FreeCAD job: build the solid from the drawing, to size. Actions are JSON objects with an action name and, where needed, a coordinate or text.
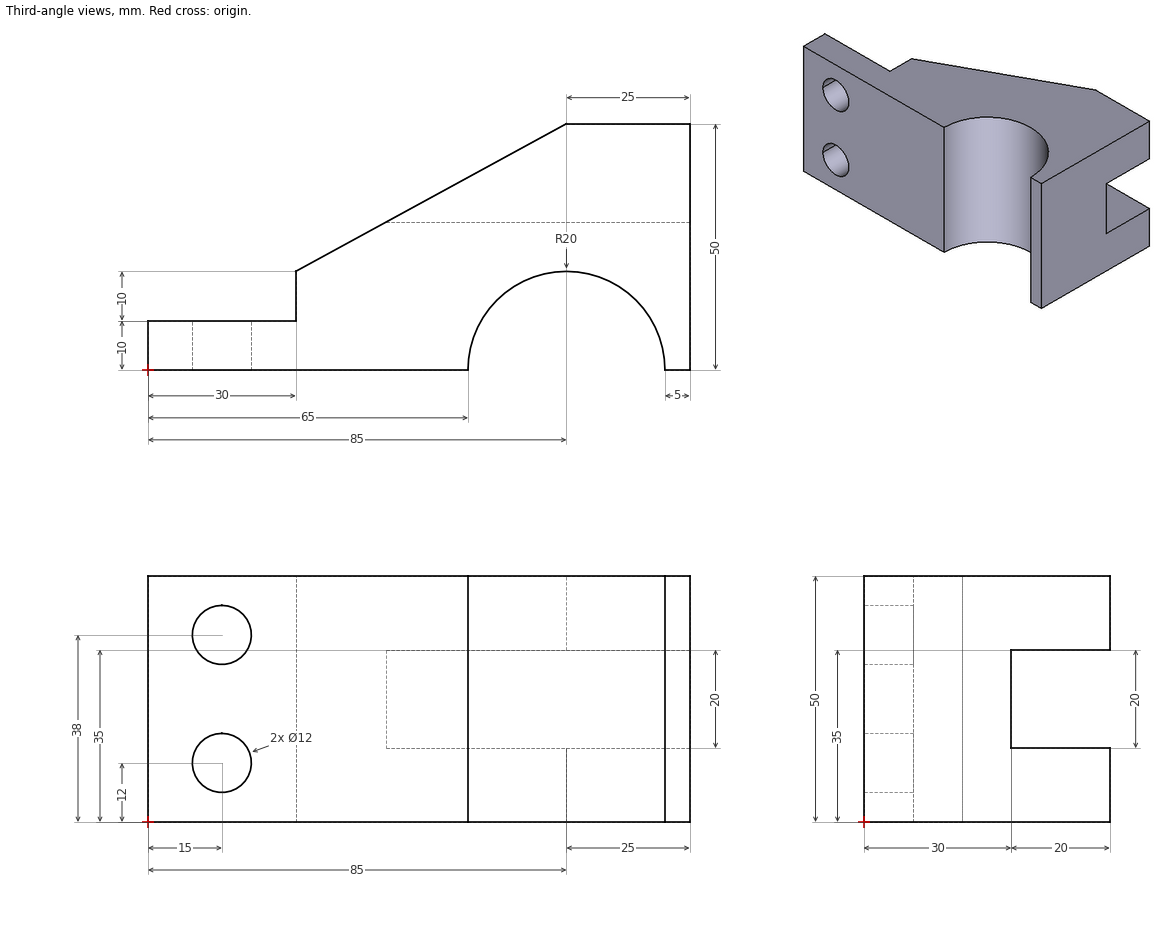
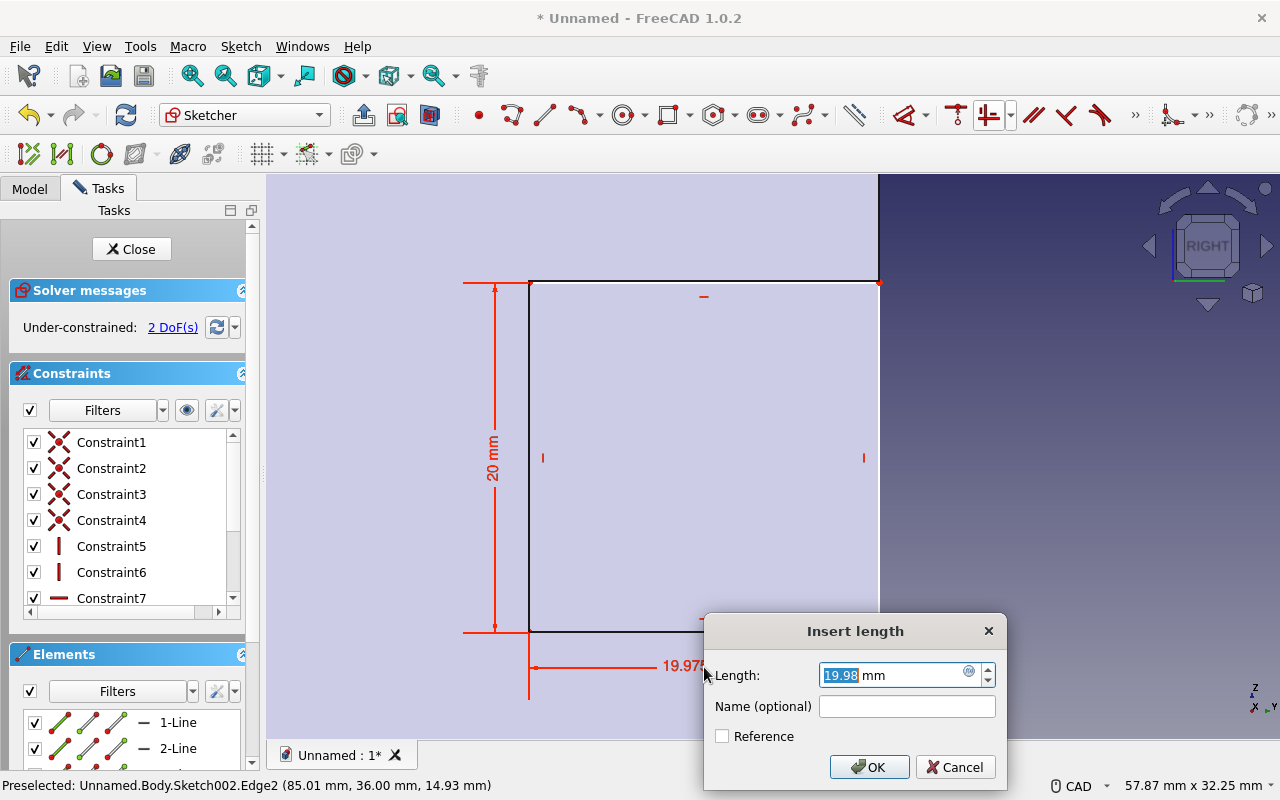
{"action": "type", "text": "20"}
{"action": "key", "text": "Return"}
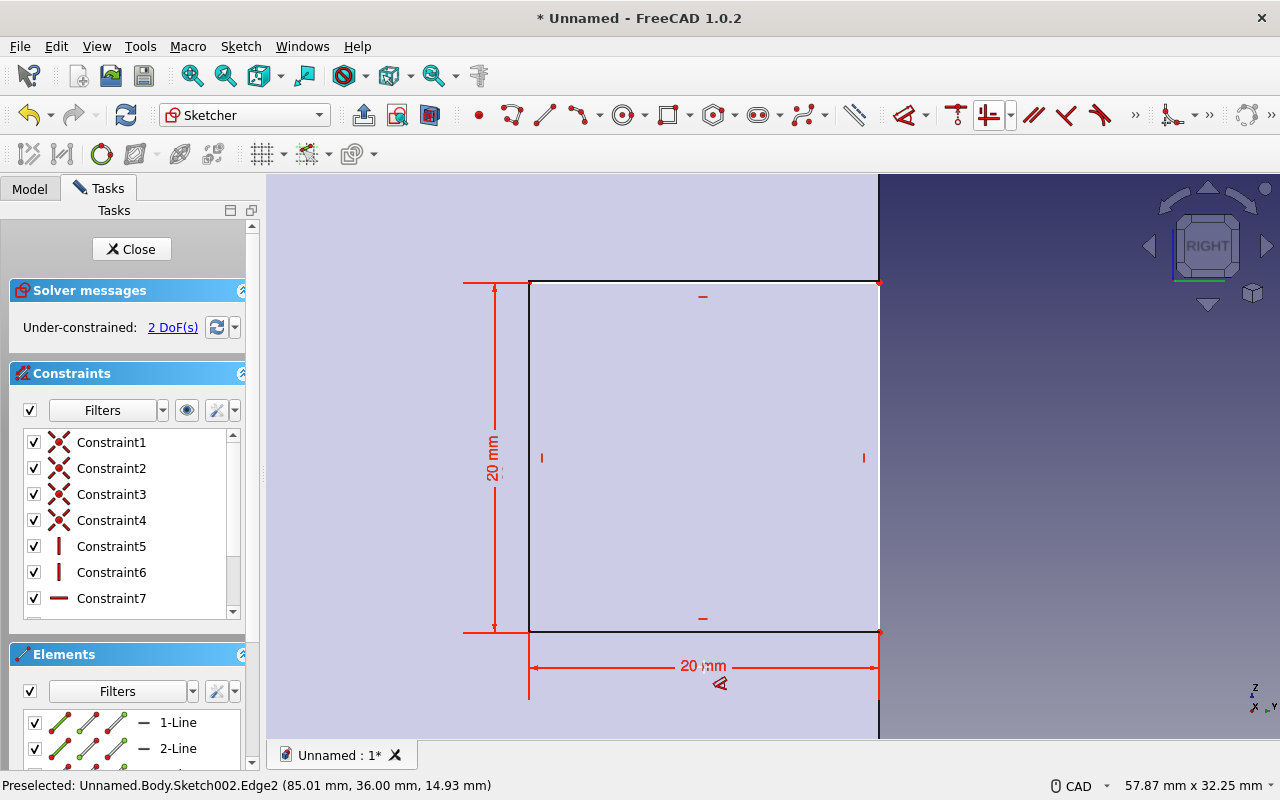
{"action": "left_click", "coordinate": [529, 283]}
{"action": "left_click", "coordinate": [411, 249]}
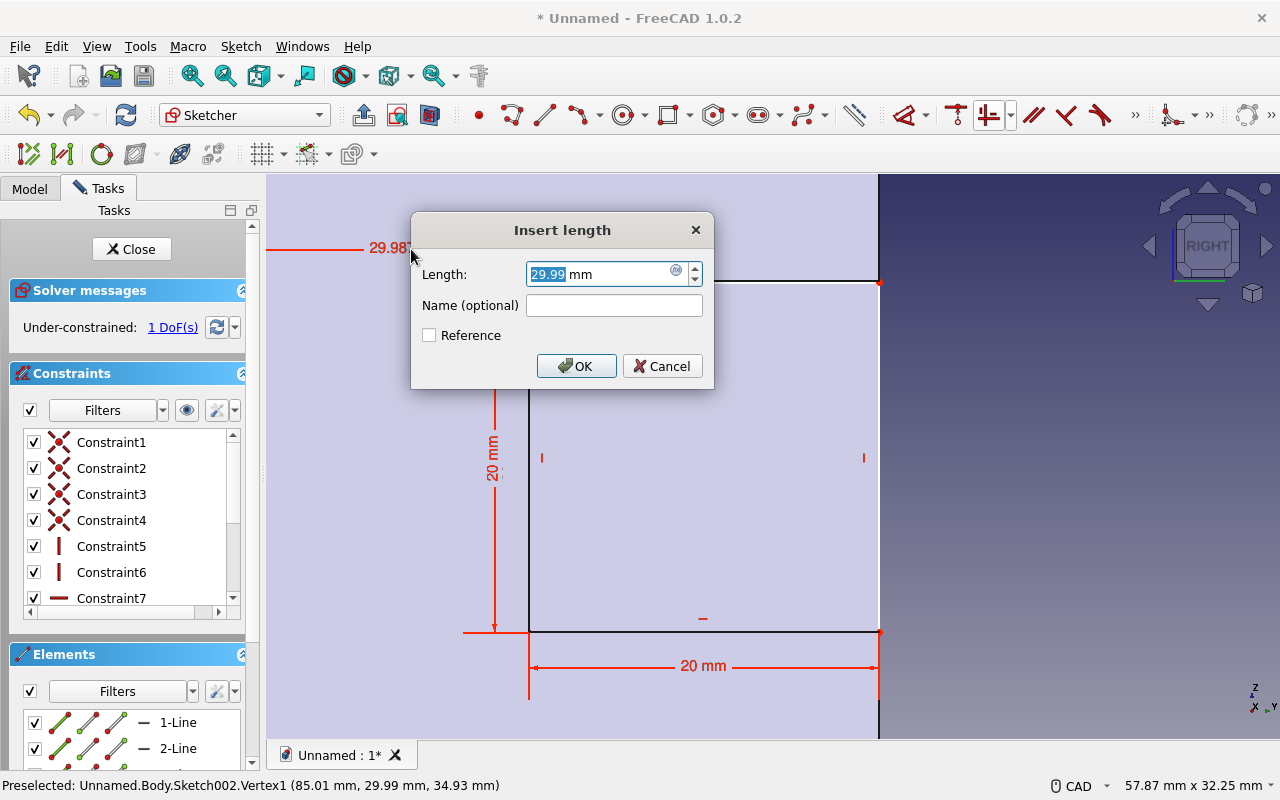
{"action": "type", "text": "30"}
{"action": "key", "text": "Return"}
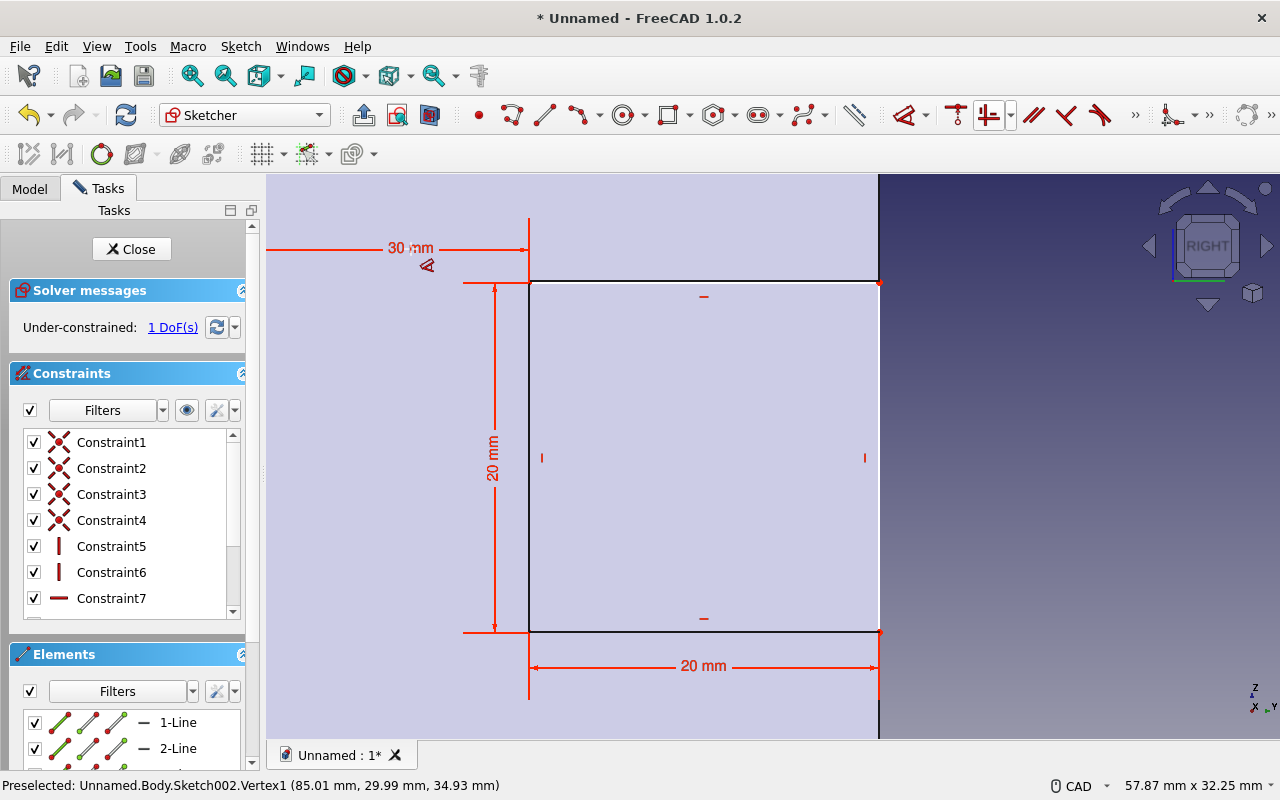
{"action": "left_click", "coordinate": [529, 283]}
{"action": "left_click", "coordinate": [563, 497]}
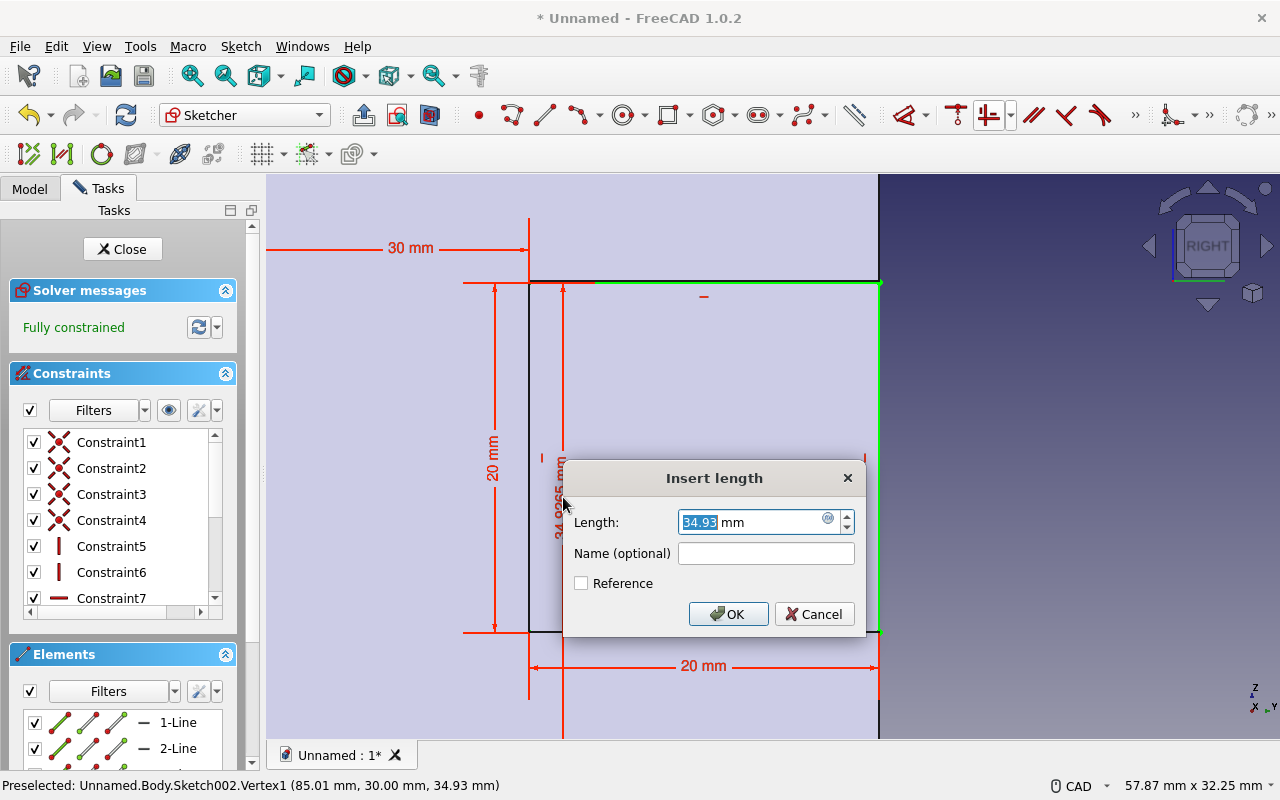
{"action": "type", "text": "35"}
{"action": "key", "text": "Return"}
{"action": "key", "text": "Escape"}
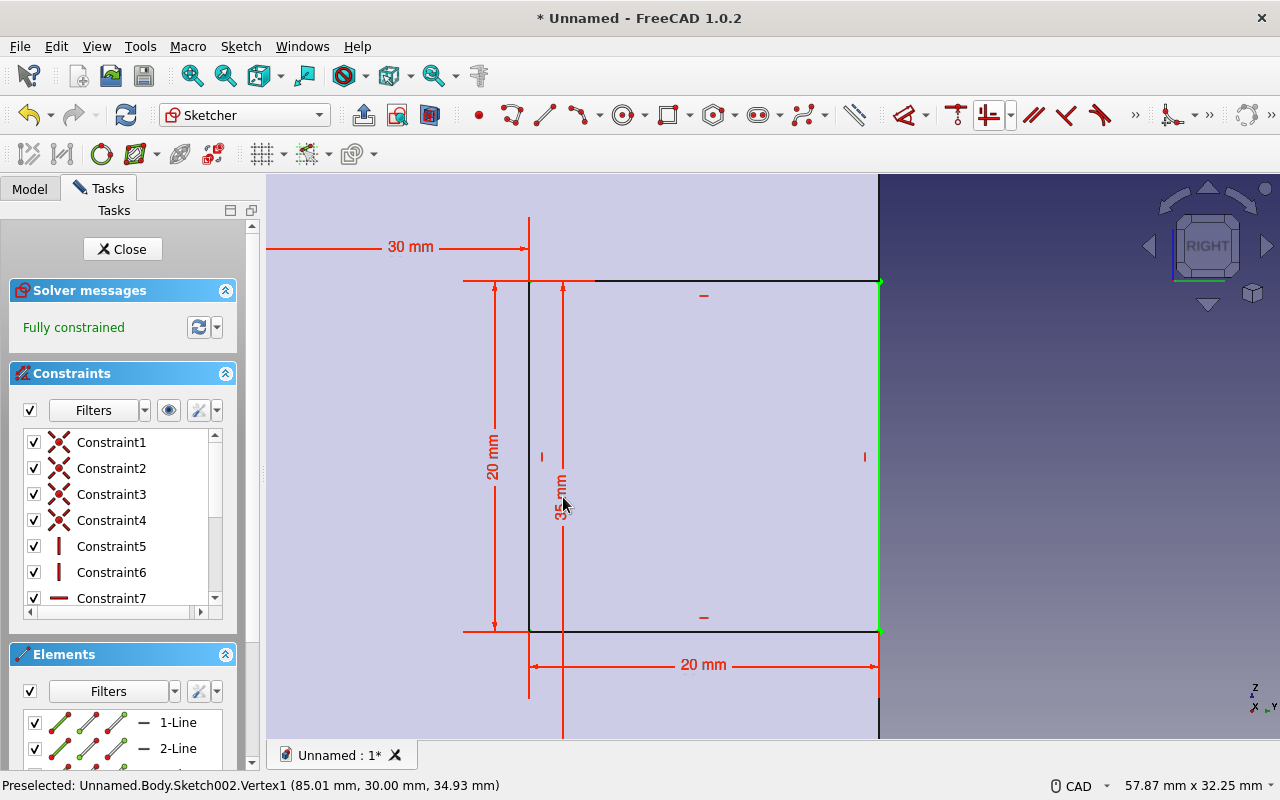
{"action": "left_click", "coordinate": [123, 249]}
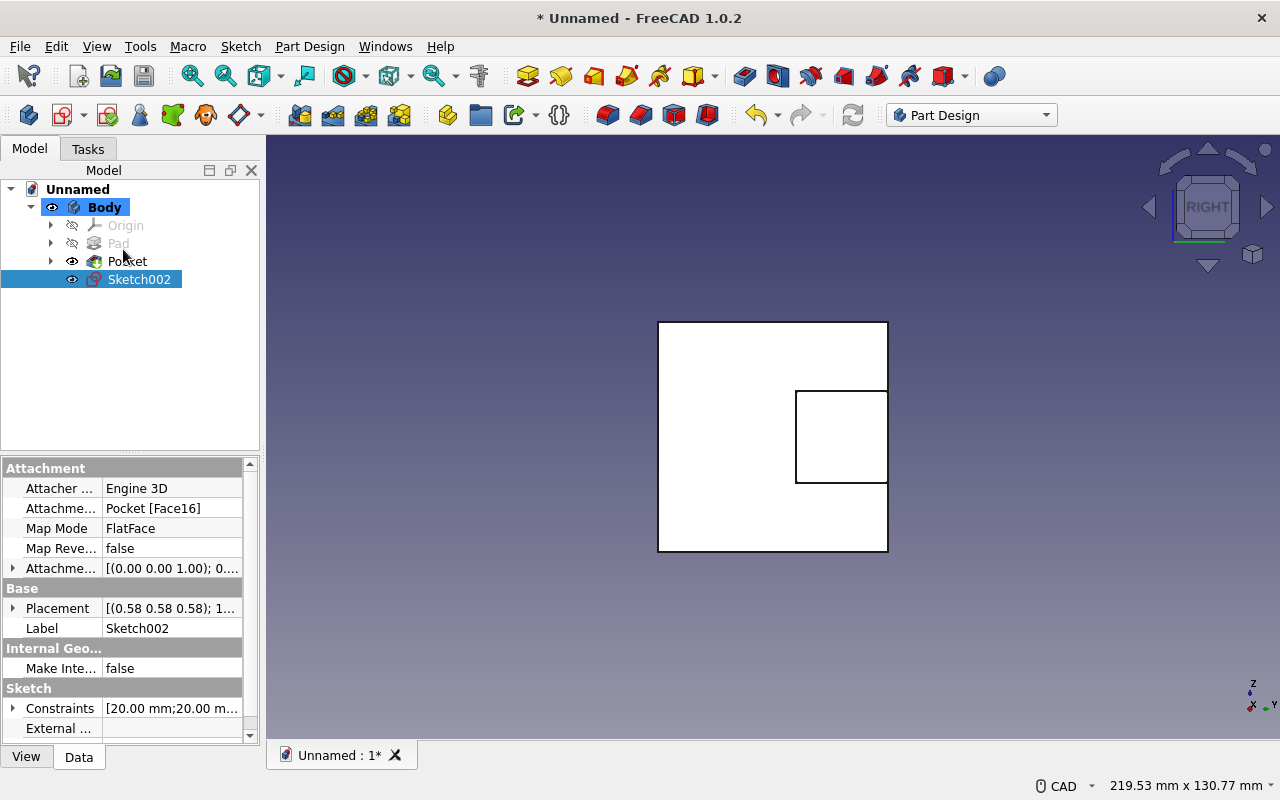
{"action": "left_click", "coordinate": [745, 76]}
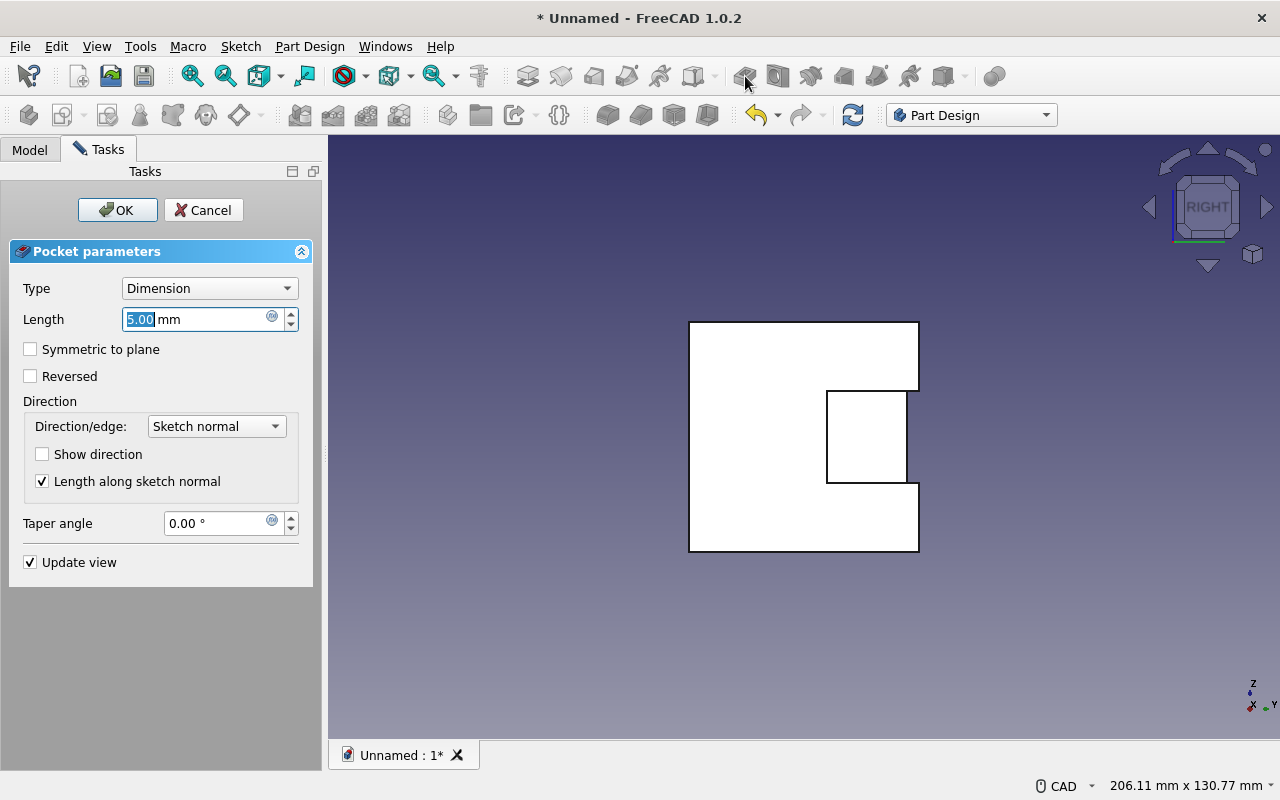
{"action": "left_click", "coordinate": [210, 288]}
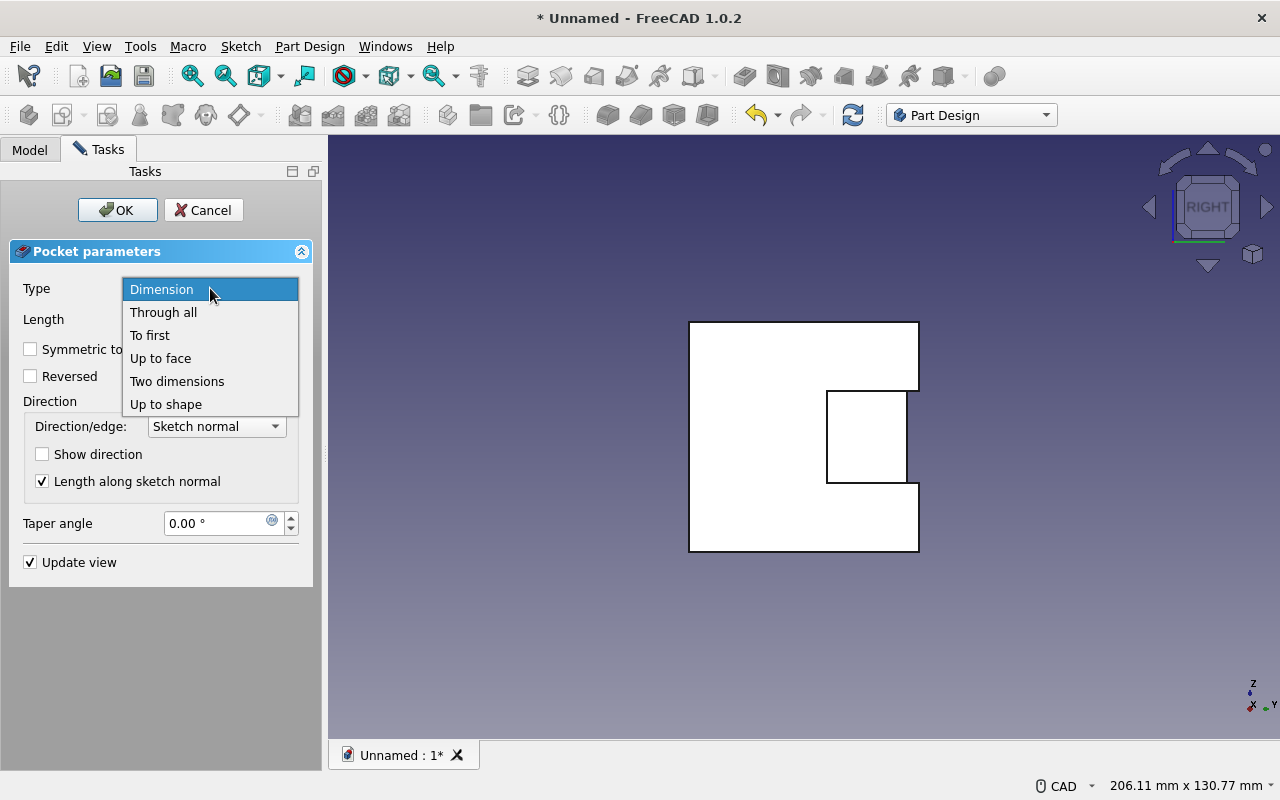
{"action": "left_click", "coordinate": [208, 312]}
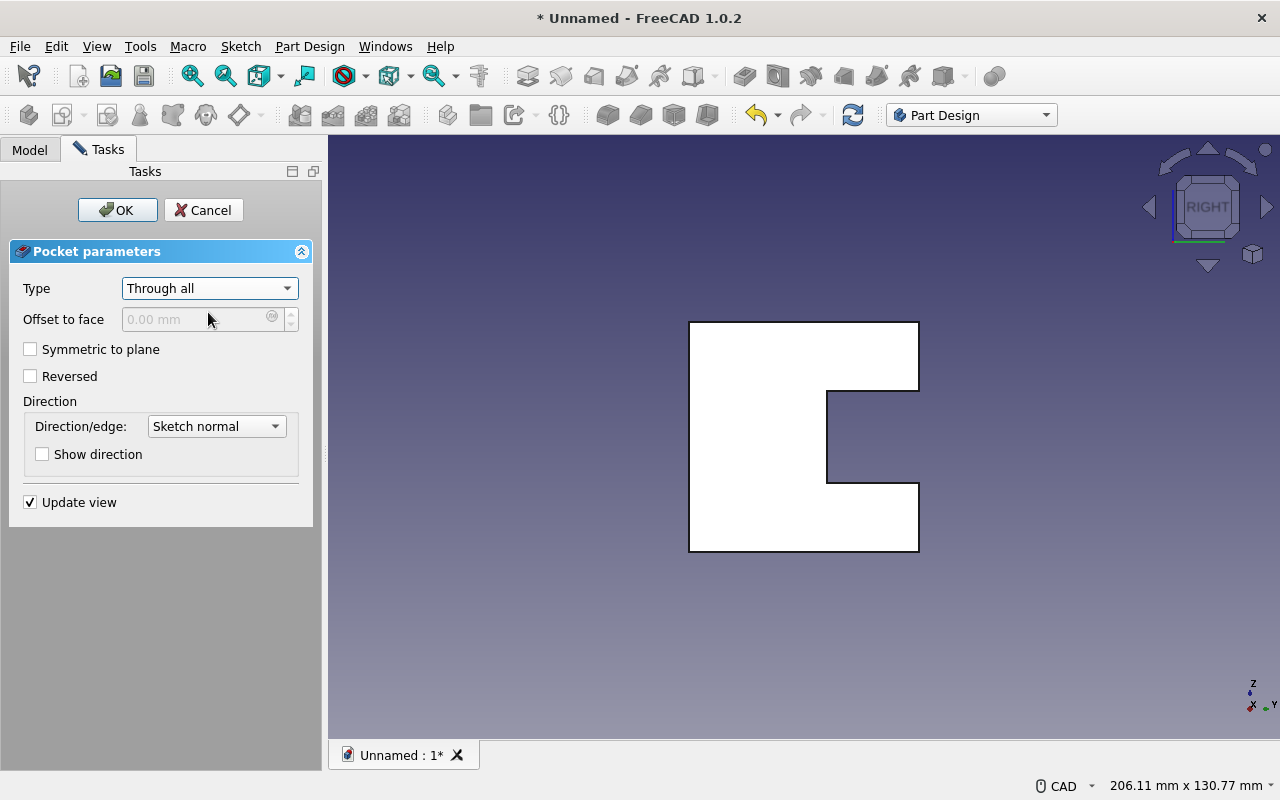
{"action": "left_click", "coordinate": [118, 210]}